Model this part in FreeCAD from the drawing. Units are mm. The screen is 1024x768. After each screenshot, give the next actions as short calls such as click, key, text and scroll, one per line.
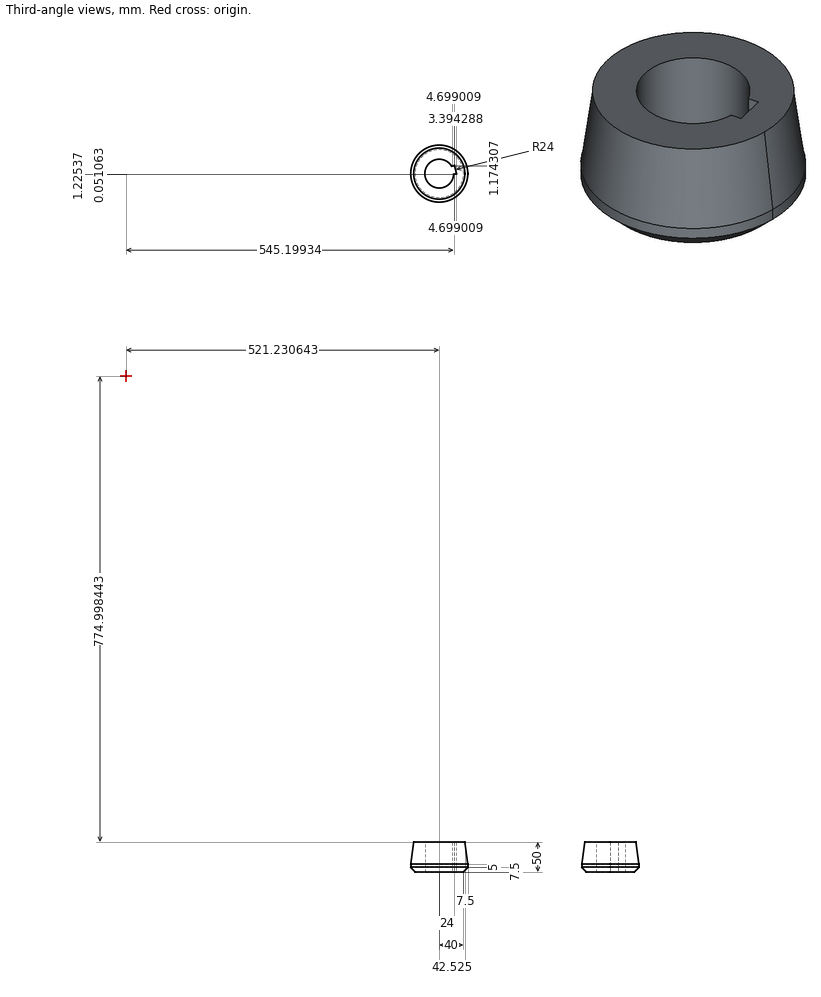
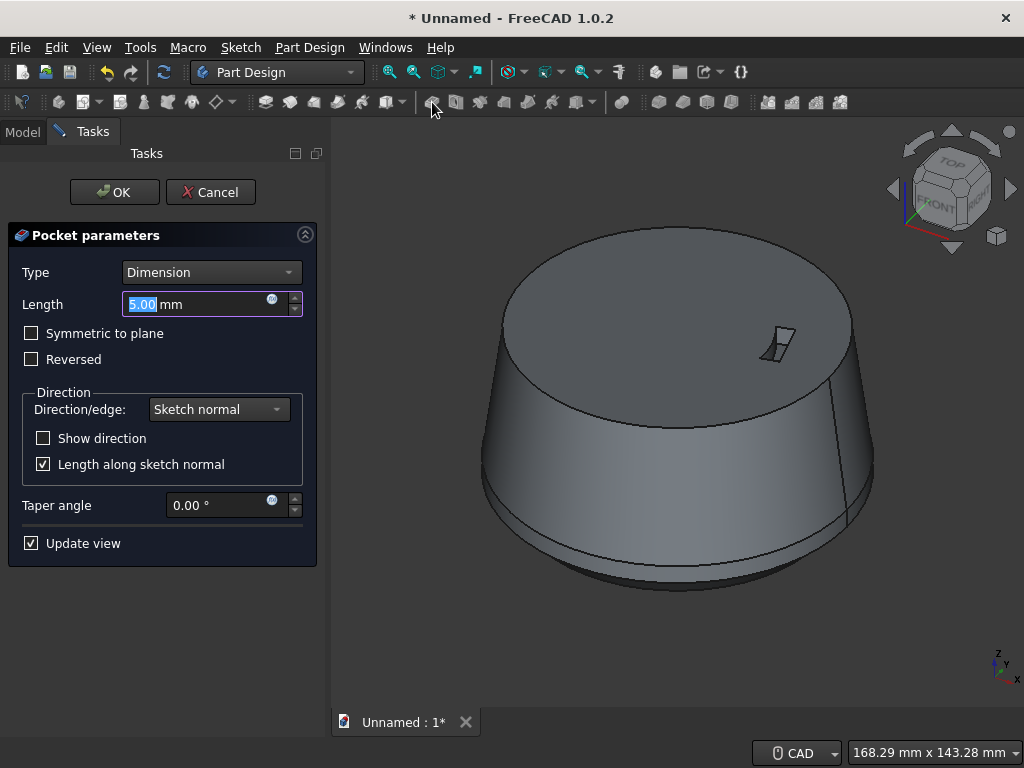
click(212, 272)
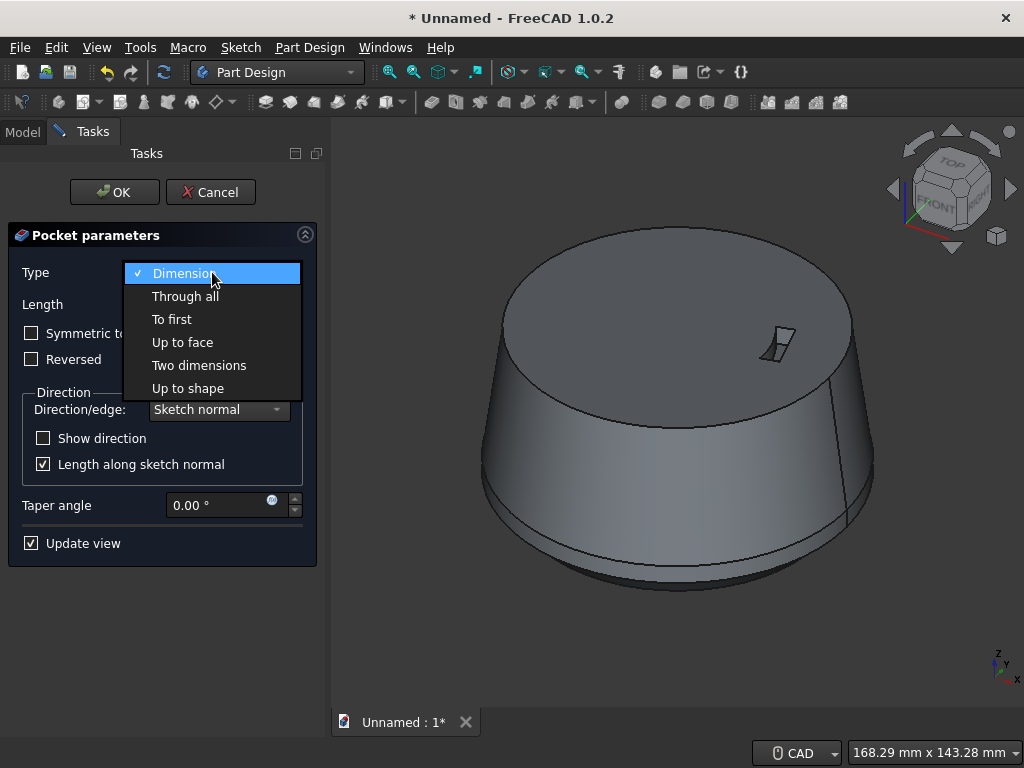
click(212, 296)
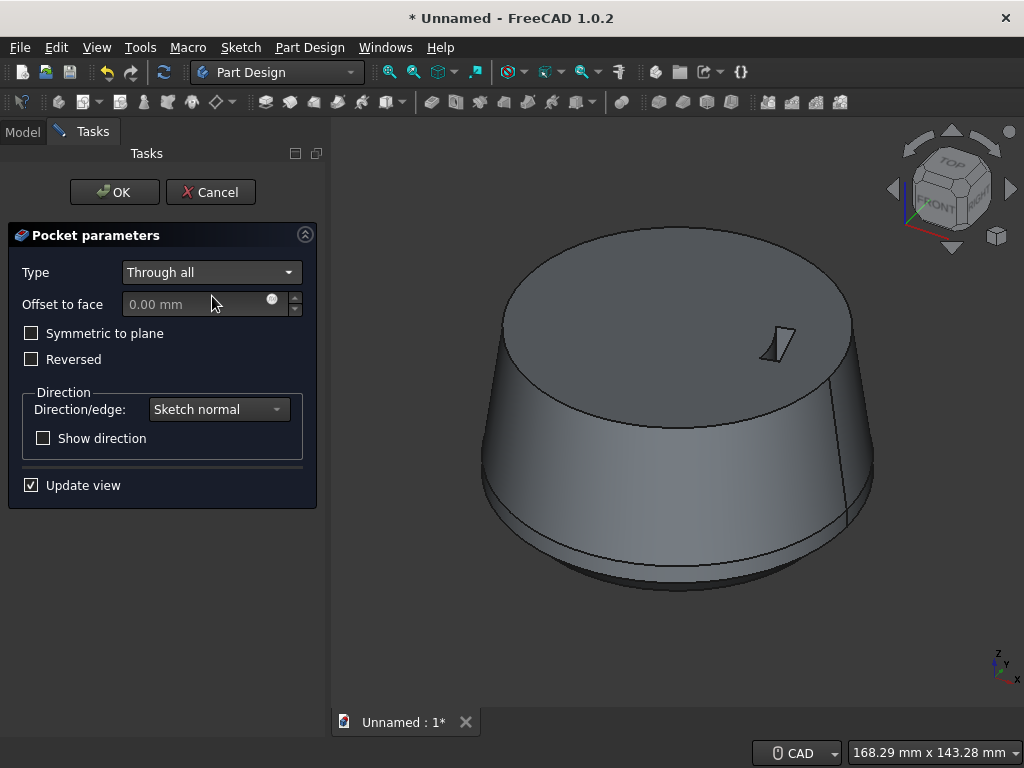
click(115, 192)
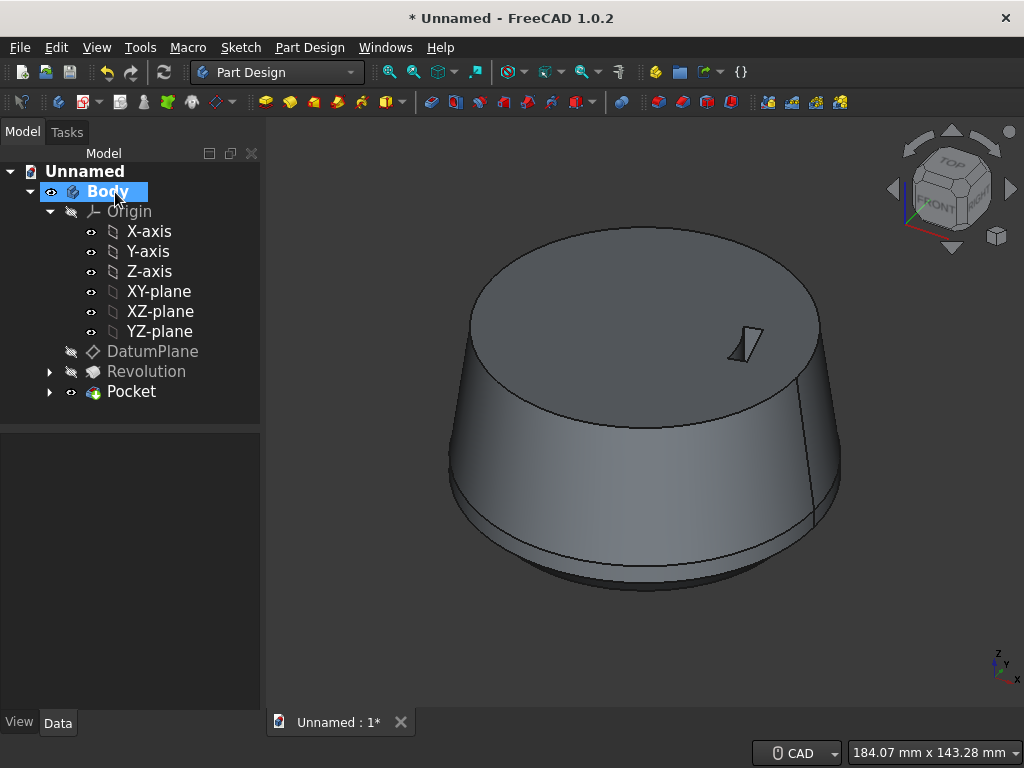
click(136, 312)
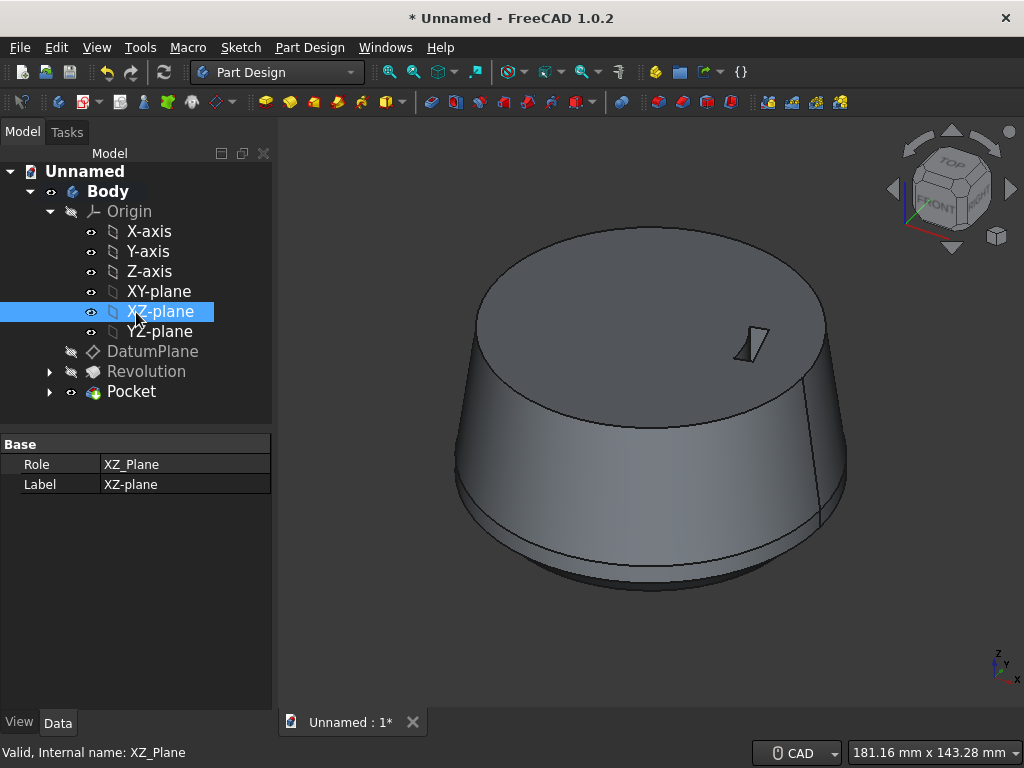
click(216, 102)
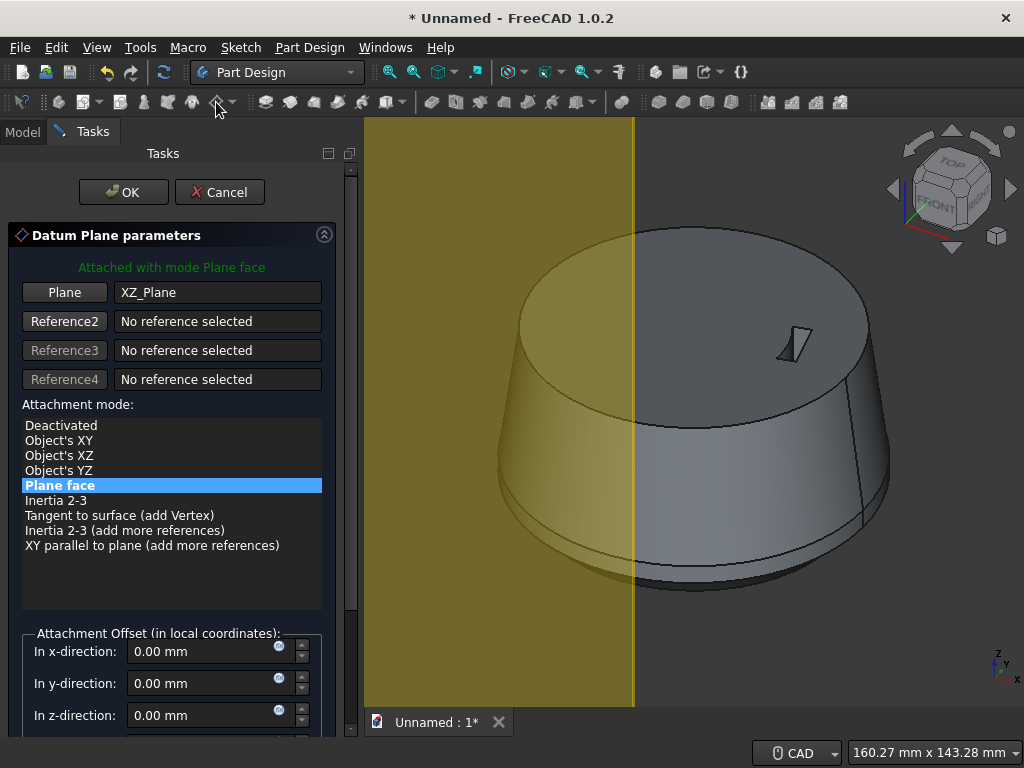
triple_click(210, 715)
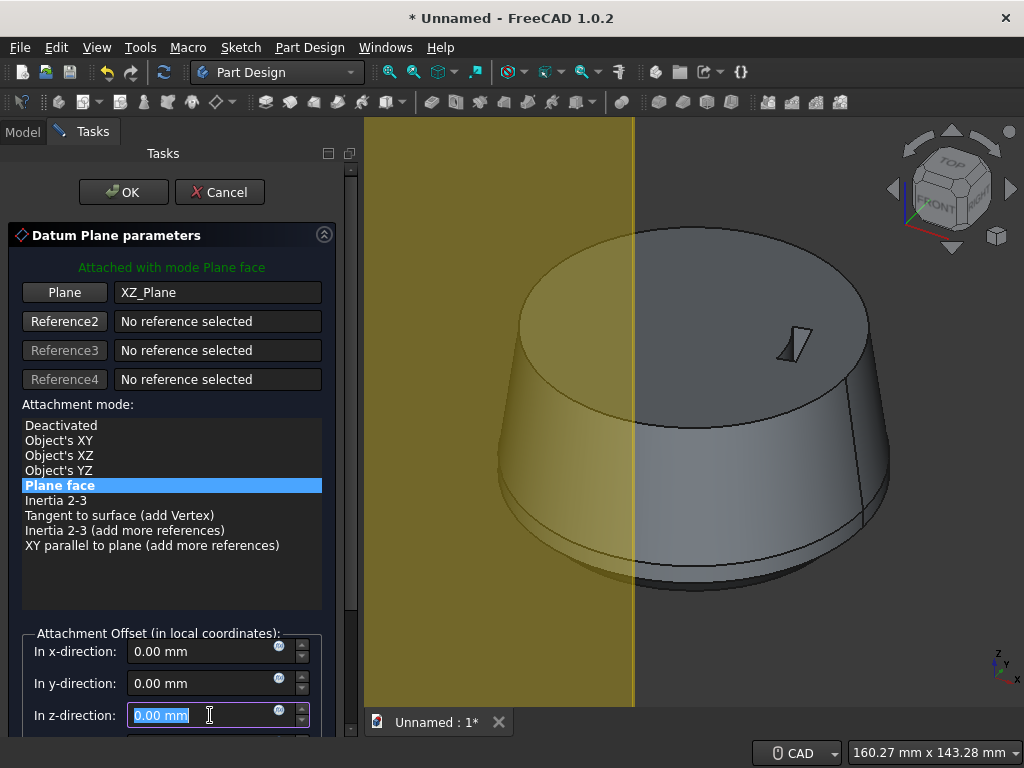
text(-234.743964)
key(Tab)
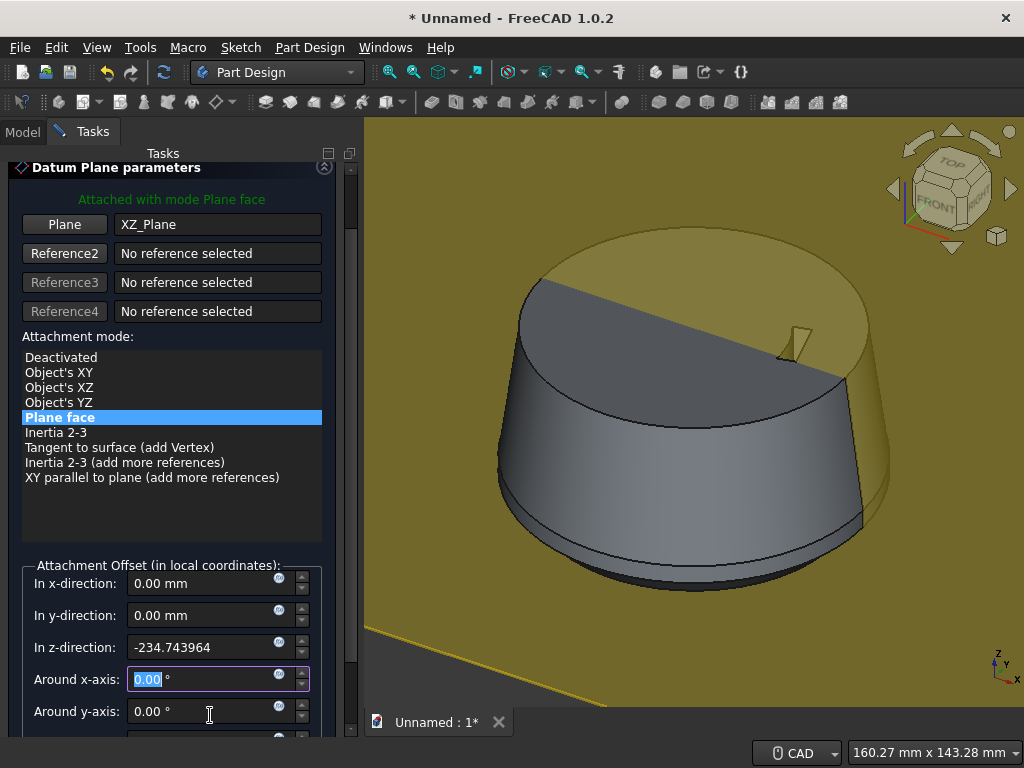
scroll(351, 450, up, 2)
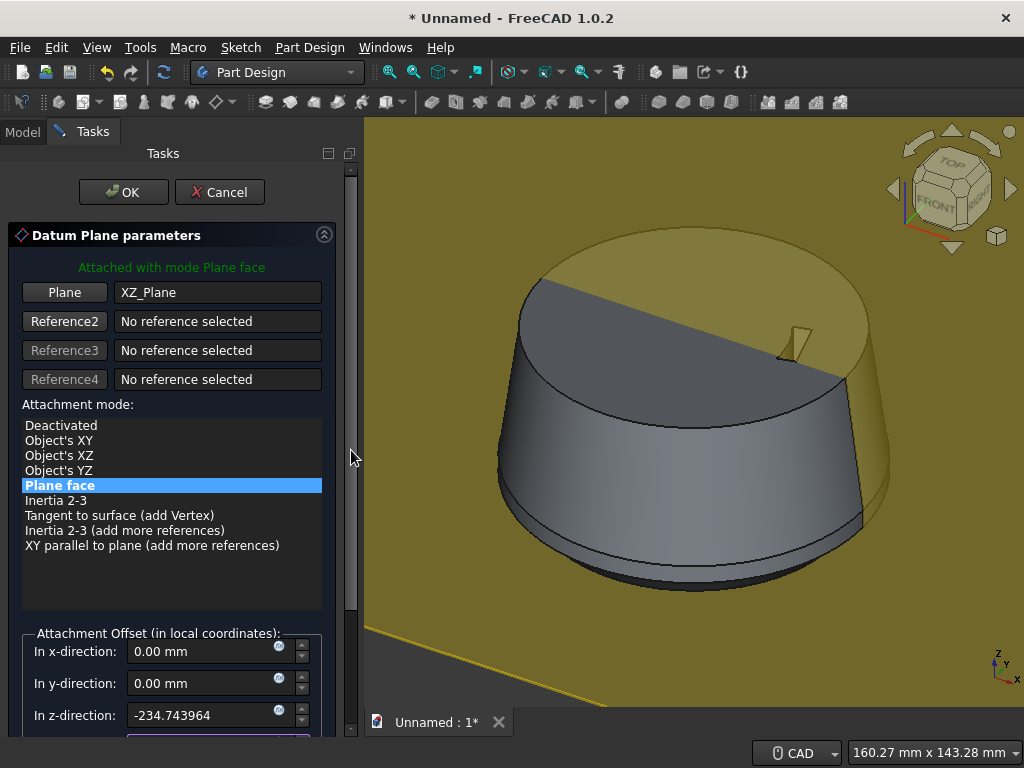
click(124, 192)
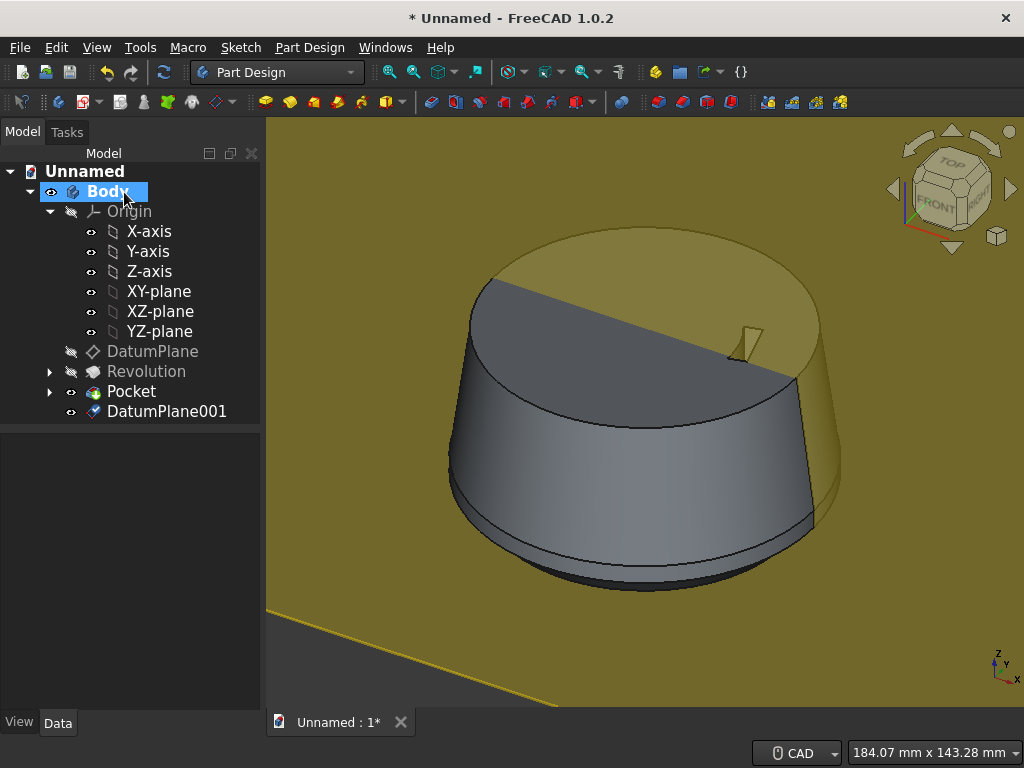
click(116, 412)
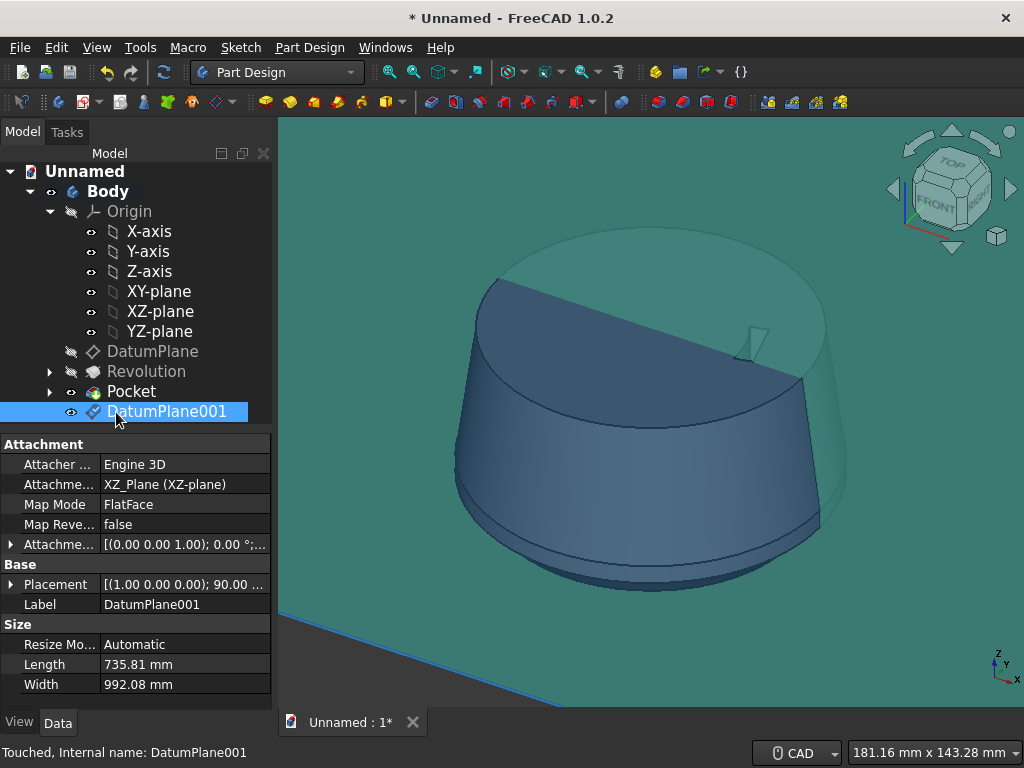
click(84, 102)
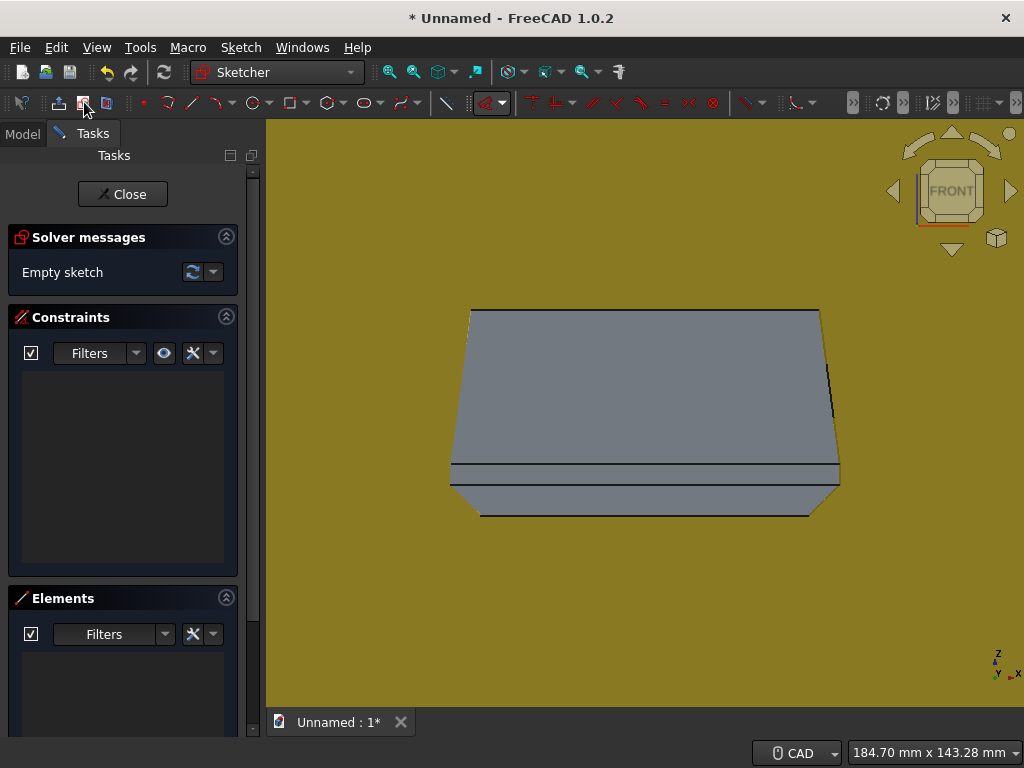
click(108, 104)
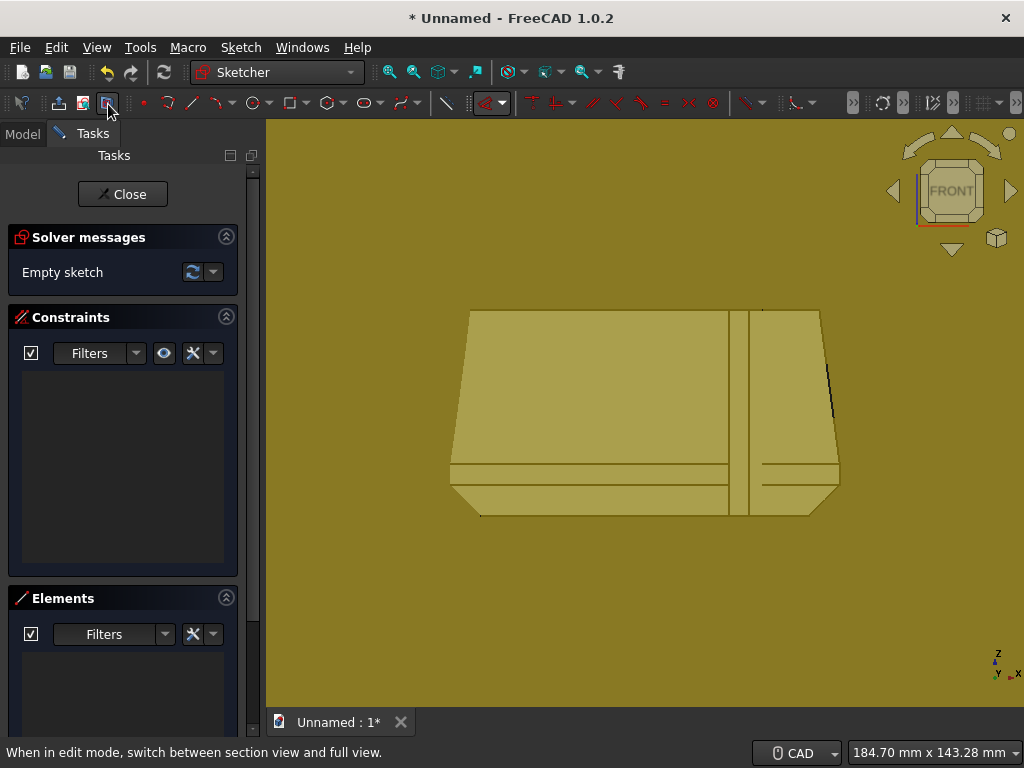
click(290, 104)